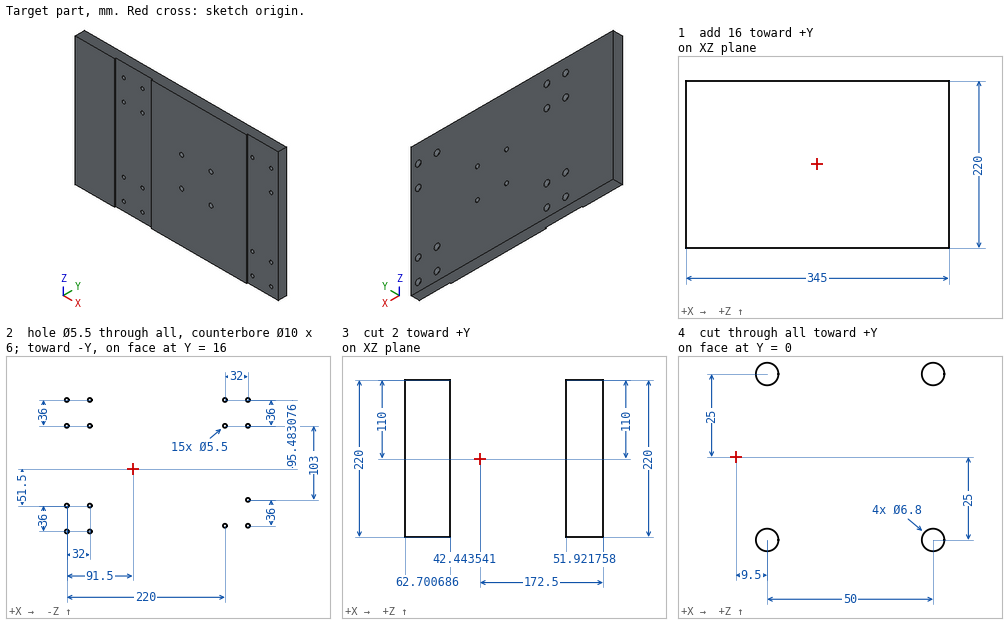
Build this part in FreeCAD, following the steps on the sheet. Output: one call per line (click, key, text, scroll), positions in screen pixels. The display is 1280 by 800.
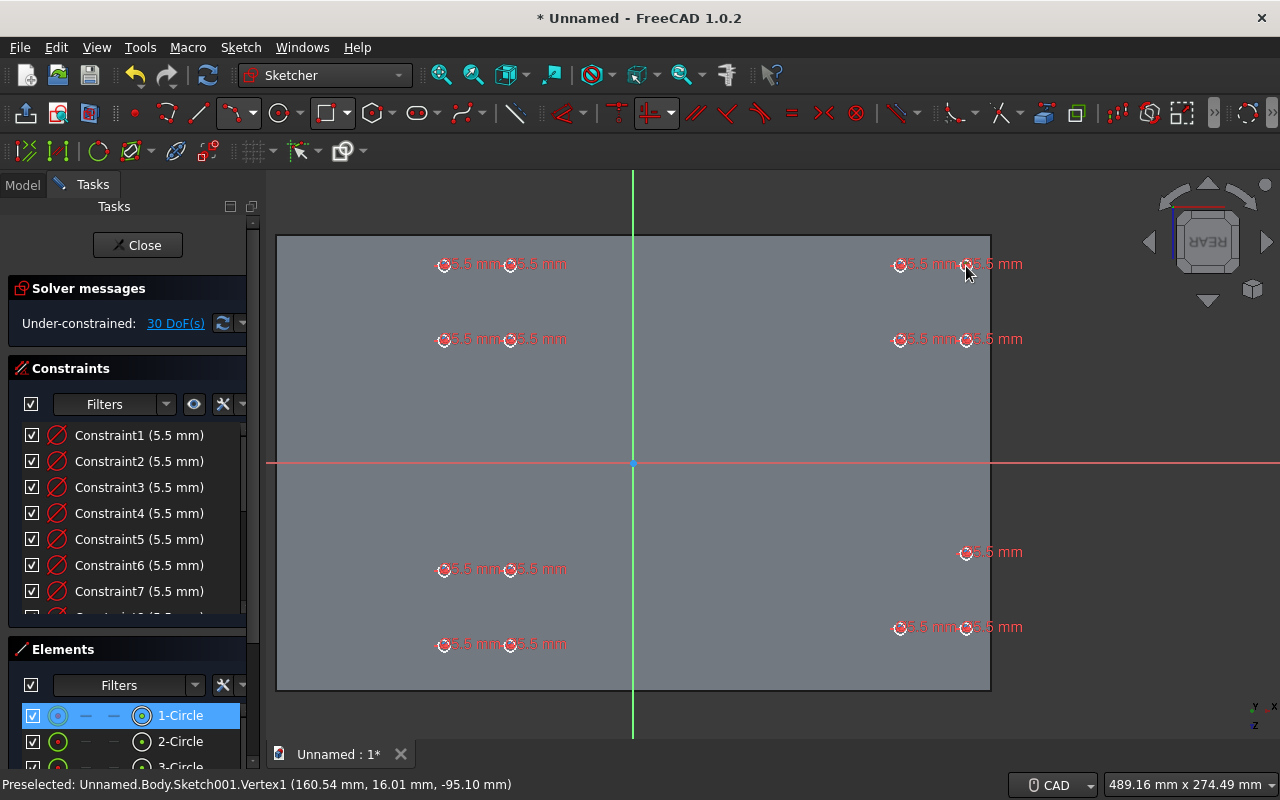
click(900, 266)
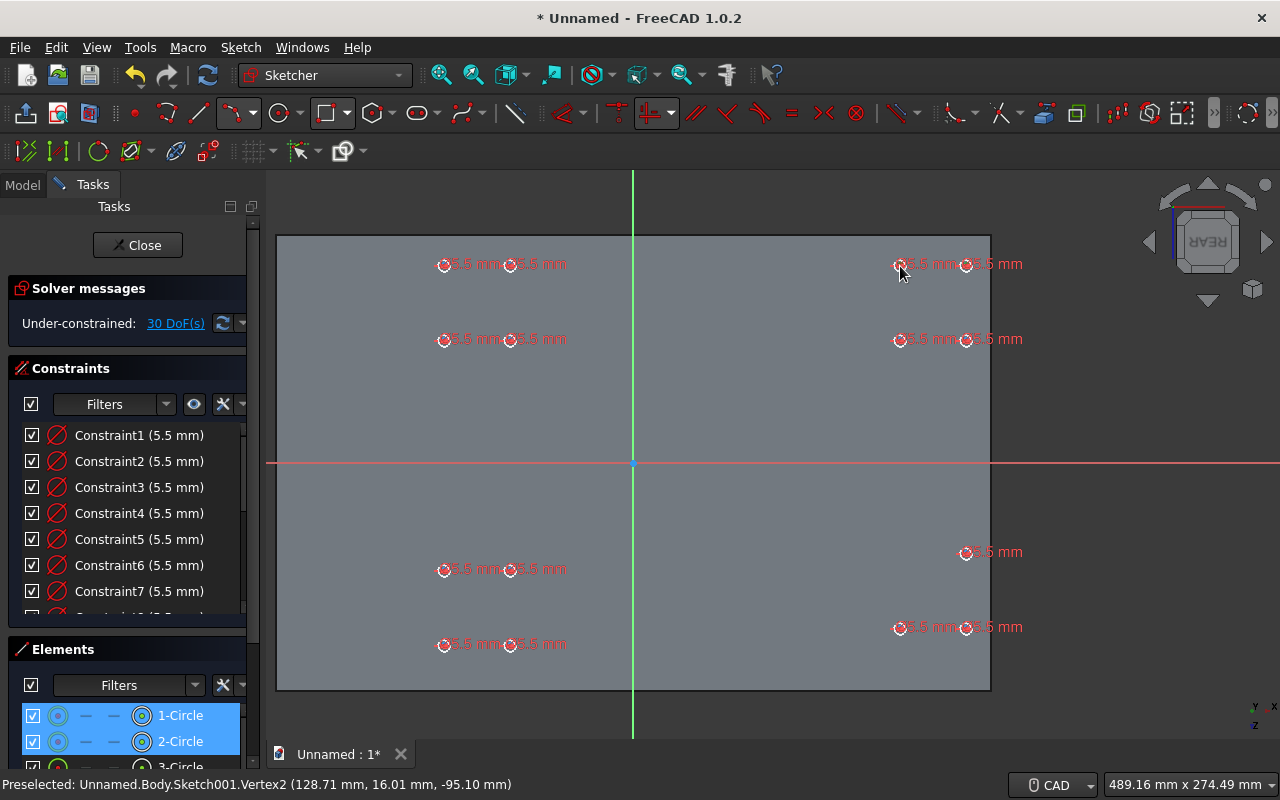
key(h)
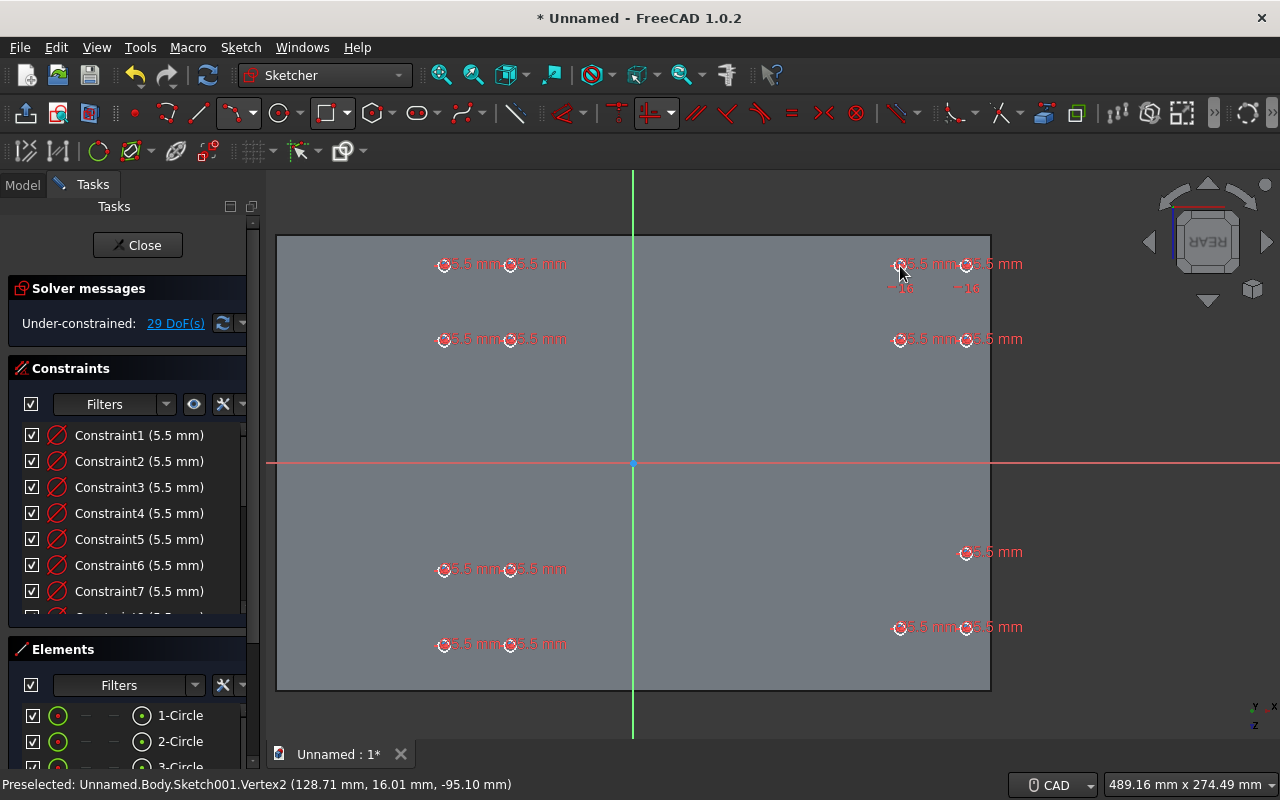
click(900, 266)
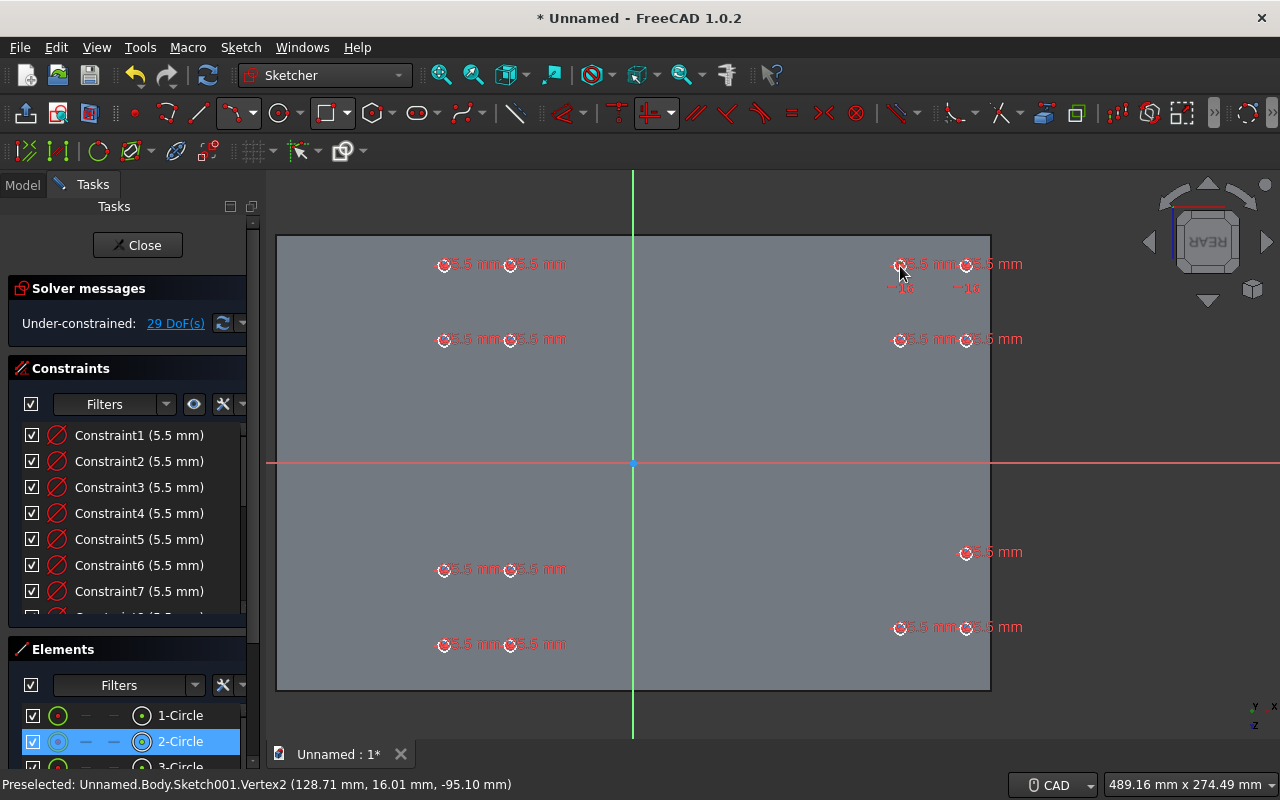
click(900, 341)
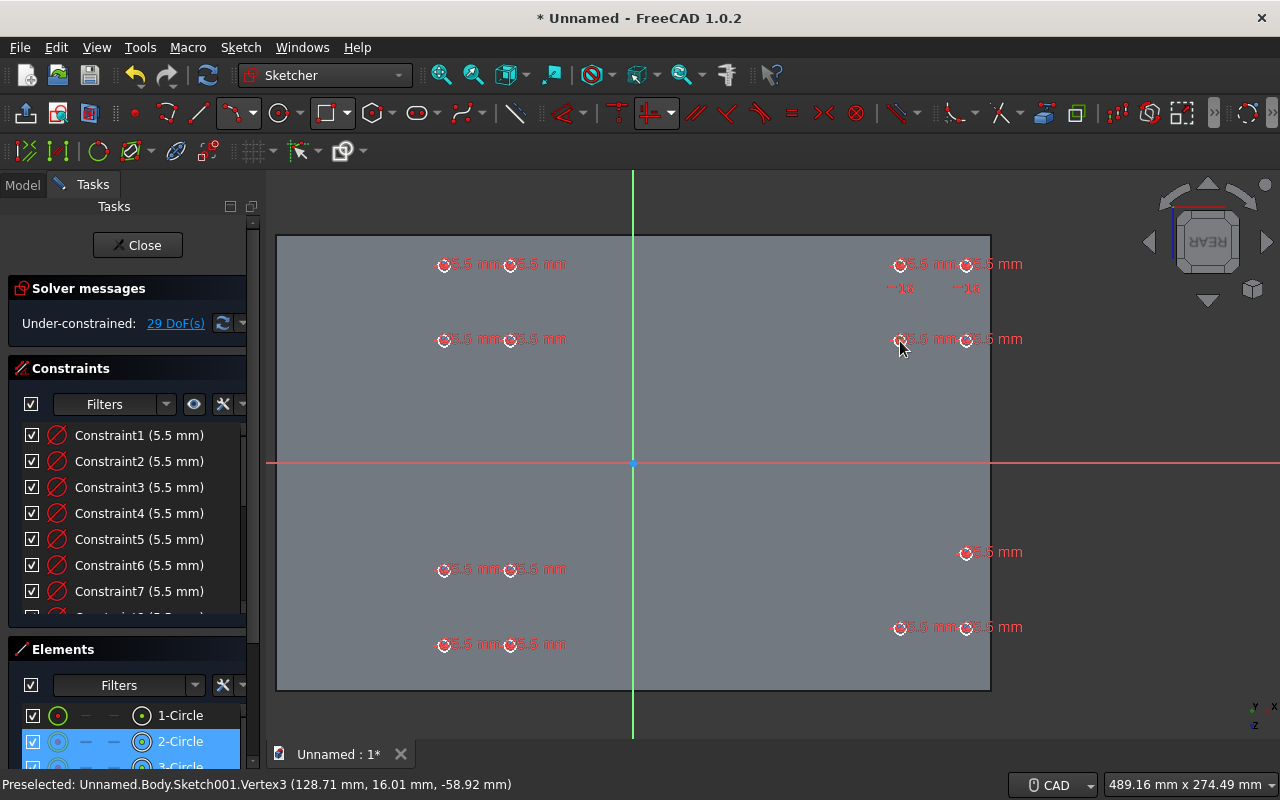
key(v)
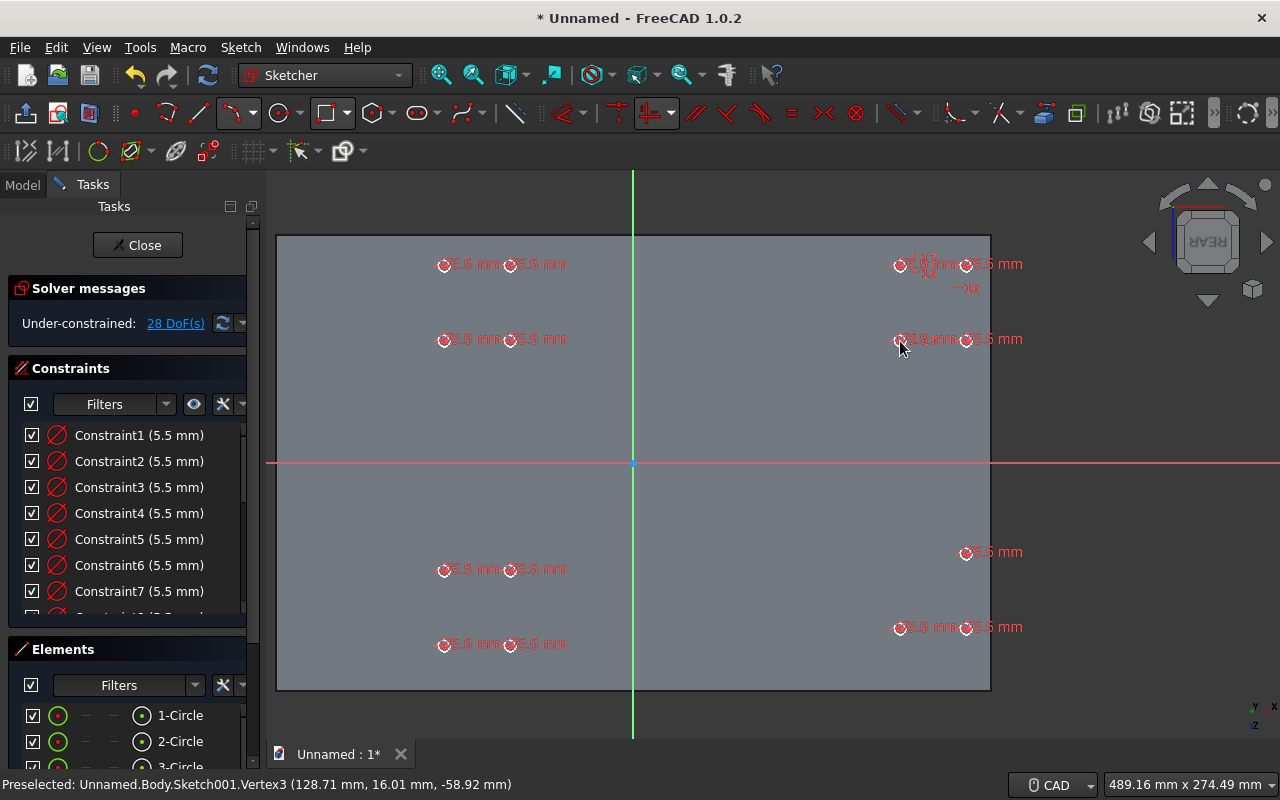
click(966, 266)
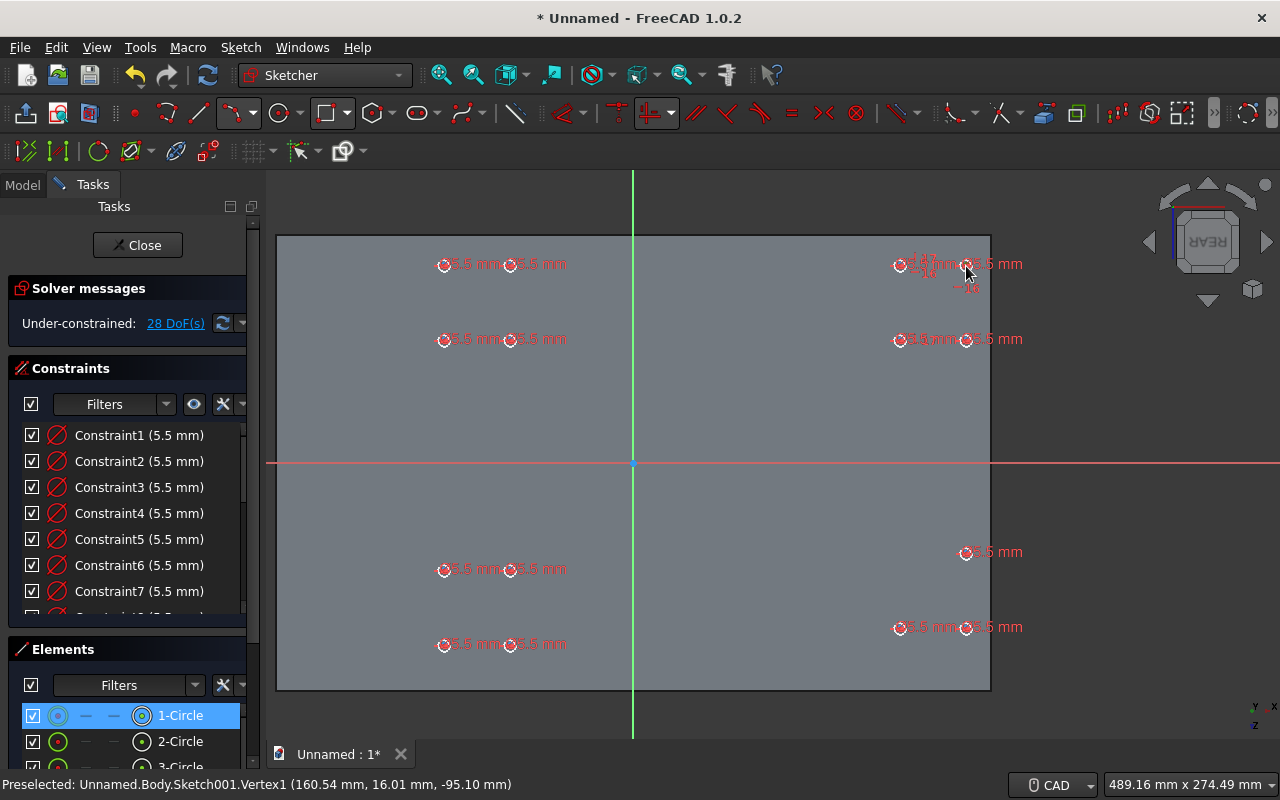
click(966, 341)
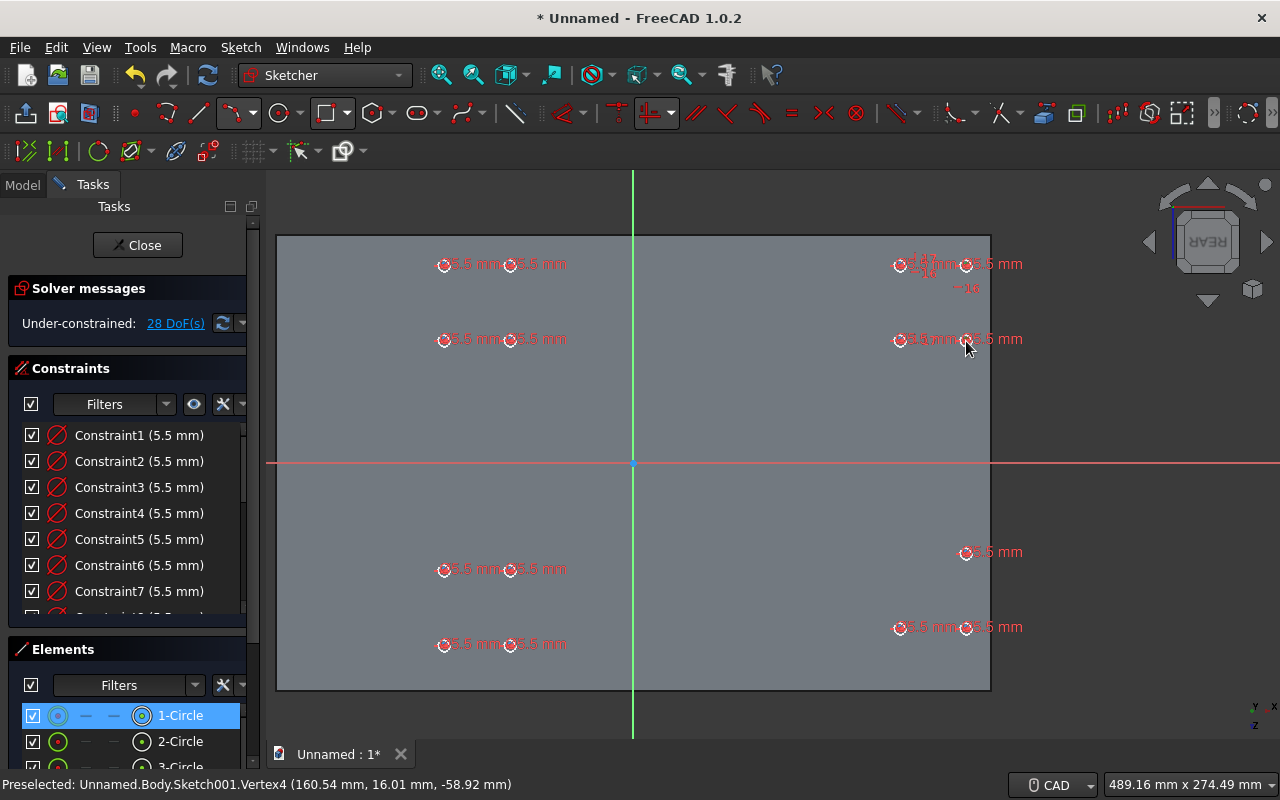
key(v)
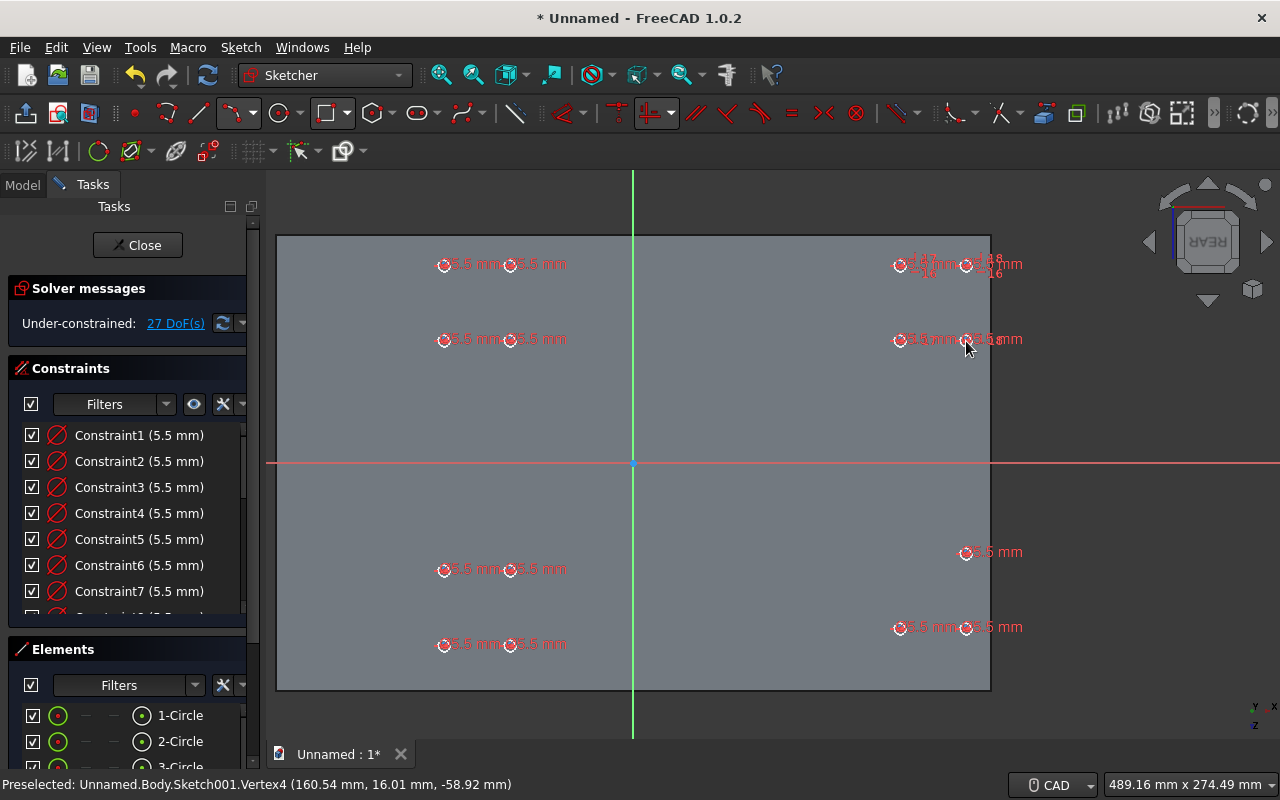
click(900, 341)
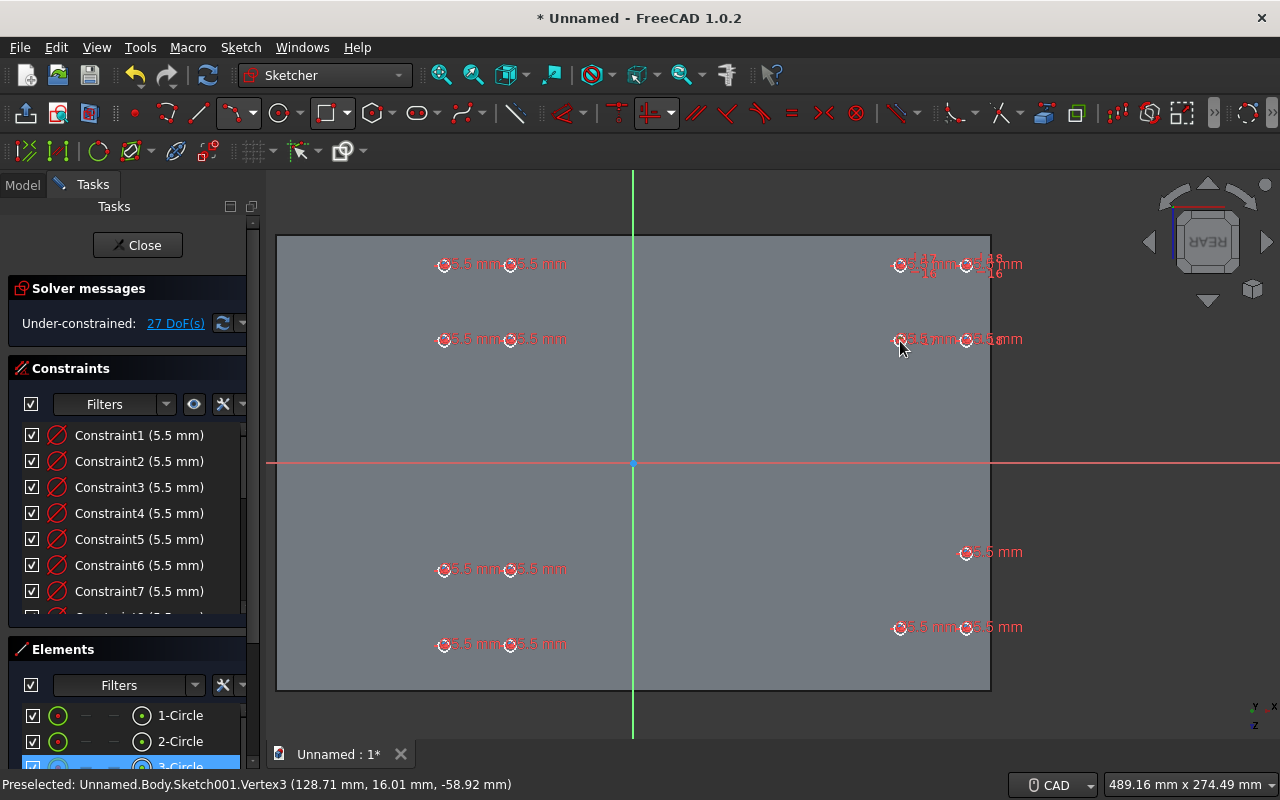
click(966, 341)